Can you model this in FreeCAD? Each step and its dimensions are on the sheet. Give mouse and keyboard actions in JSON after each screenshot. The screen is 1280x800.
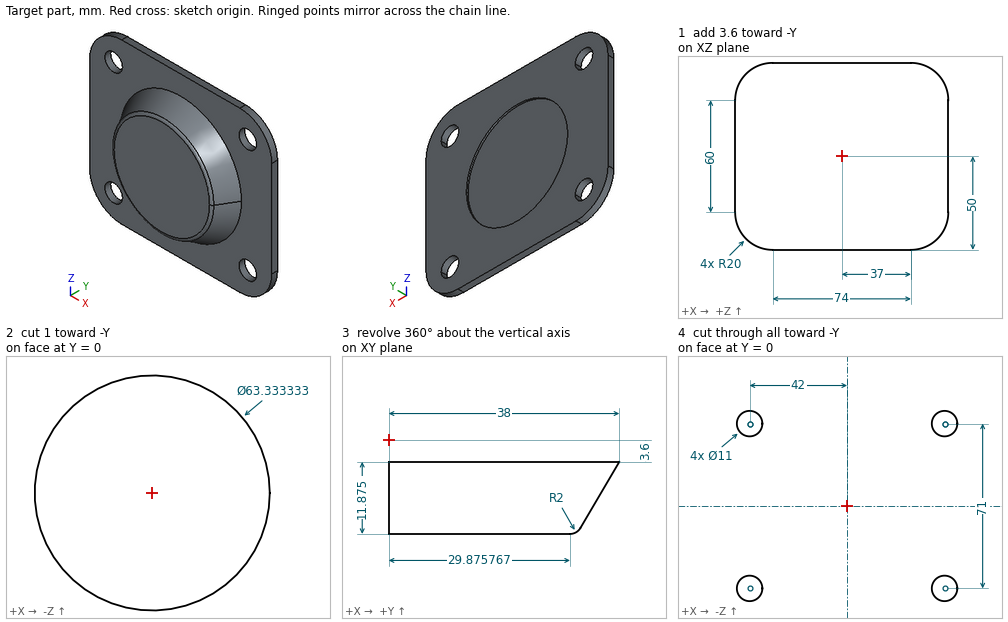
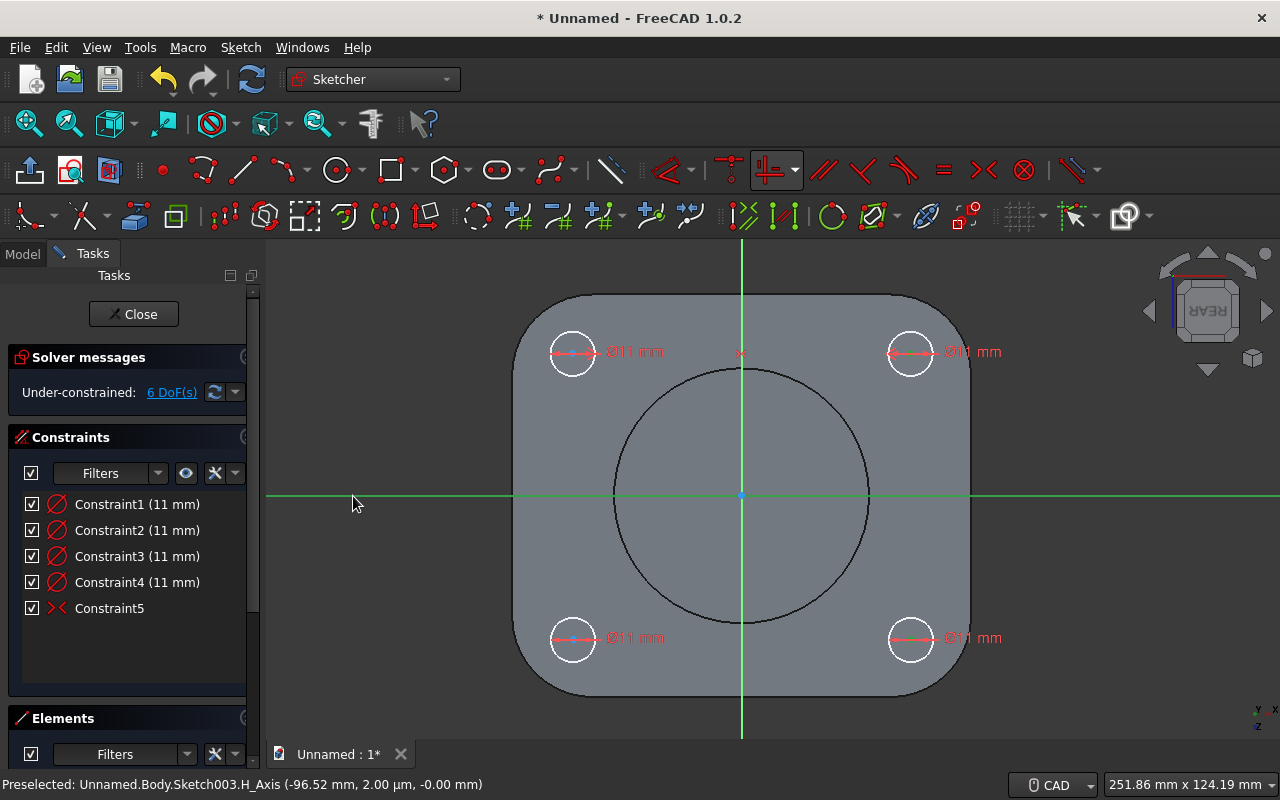
{"action": "left_click", "coordinate": [984, 170]}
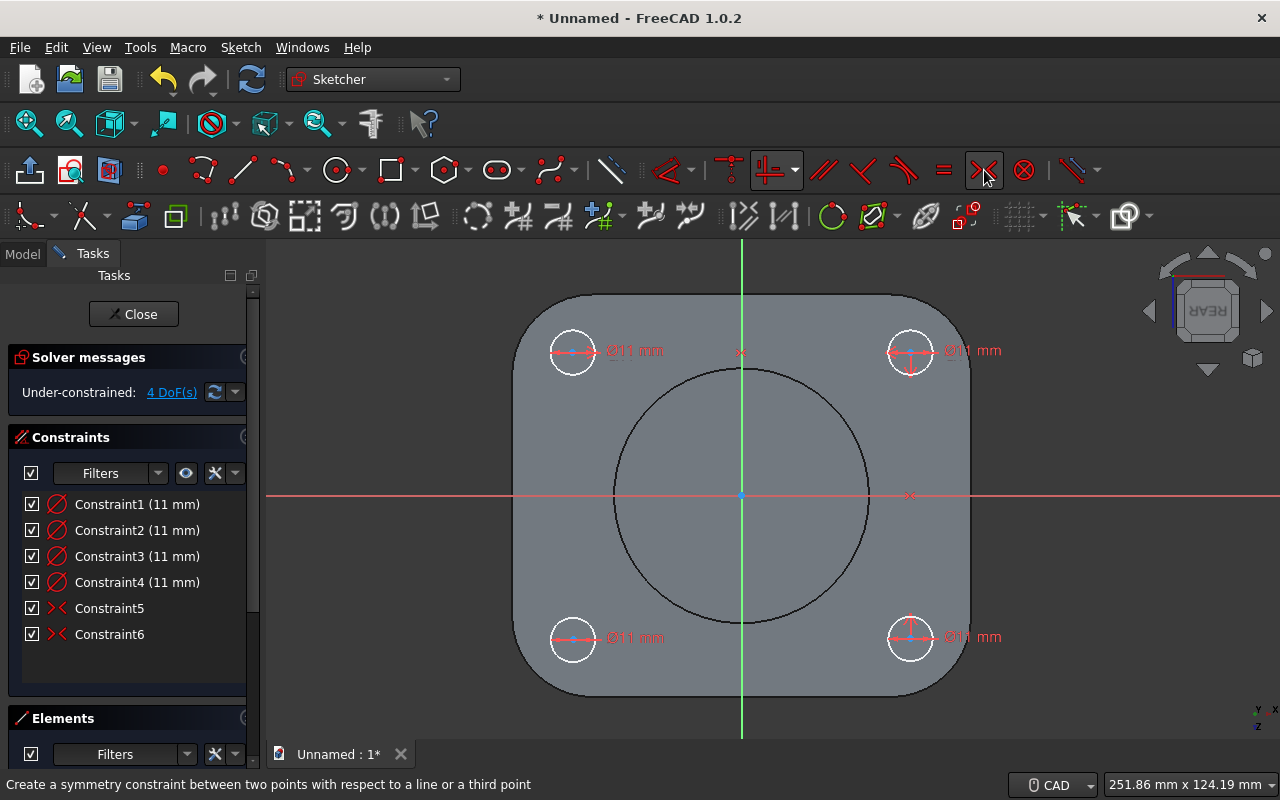
{"action": "left_click", "coordinate": [573, 353]}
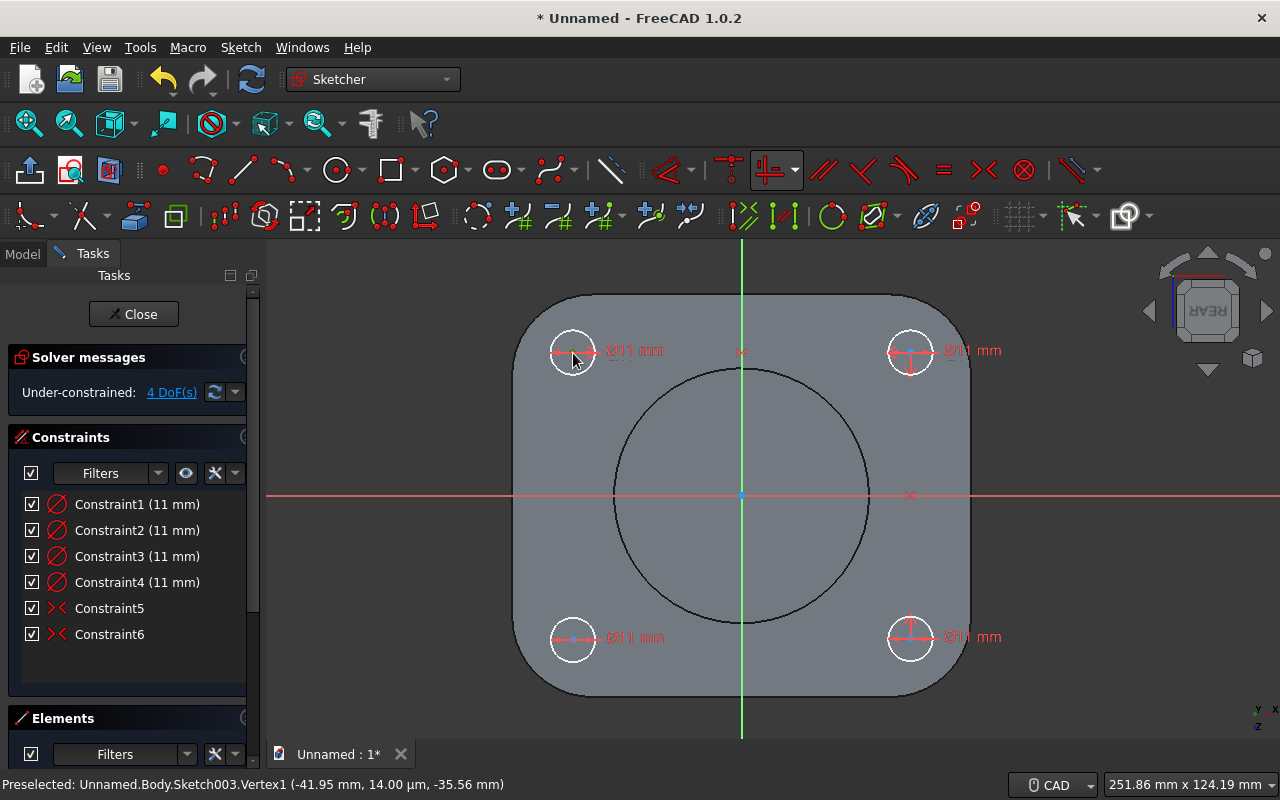
{"action": "left_click", "coordinate": [573, 640]}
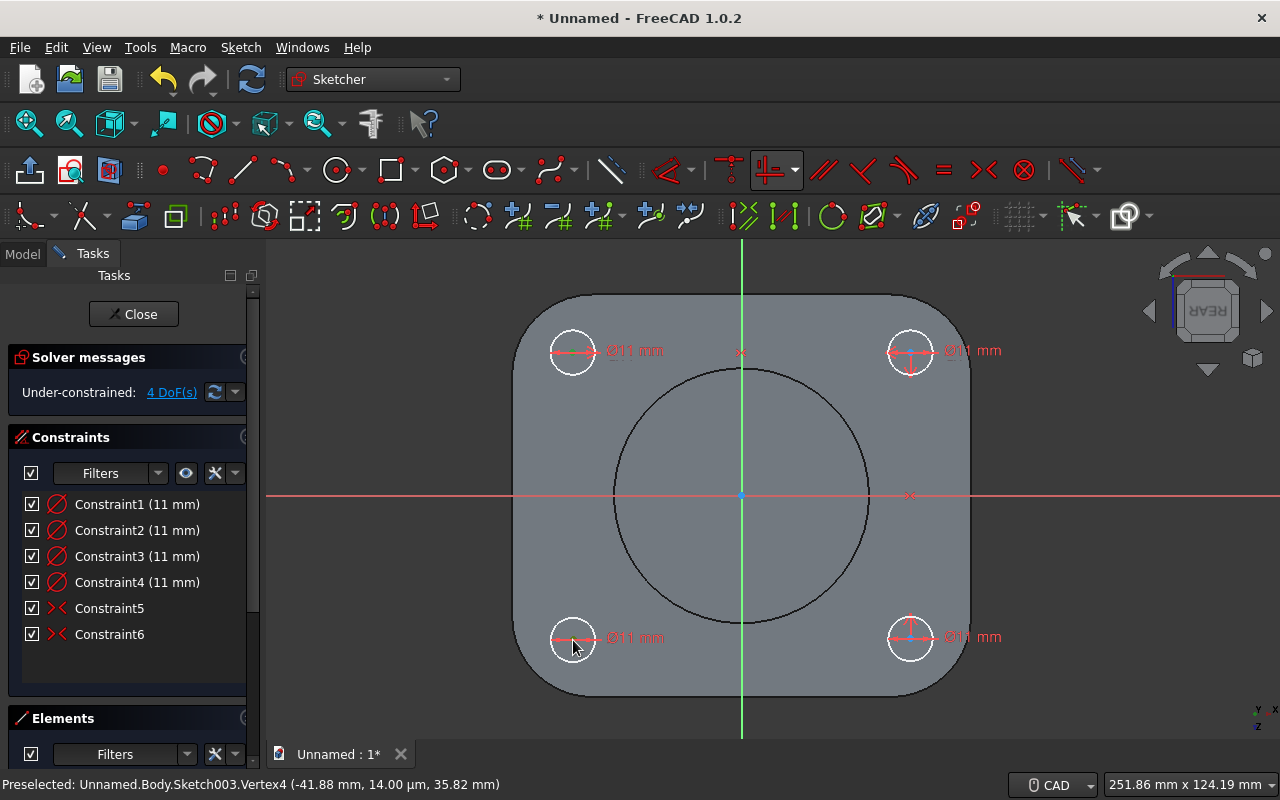
{"action": "left_click", "coordinate": [353, 496]}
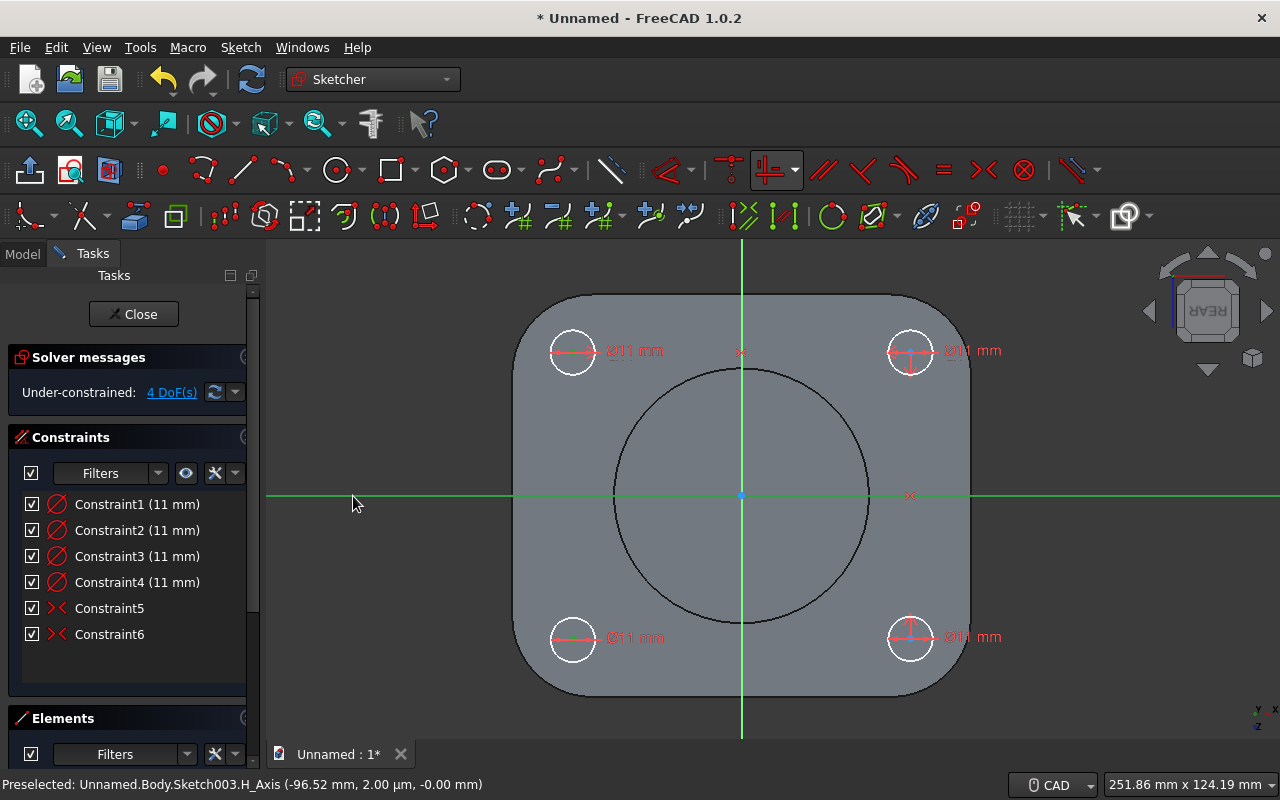
{"action": "left_click", "coordinate": [984, 170]}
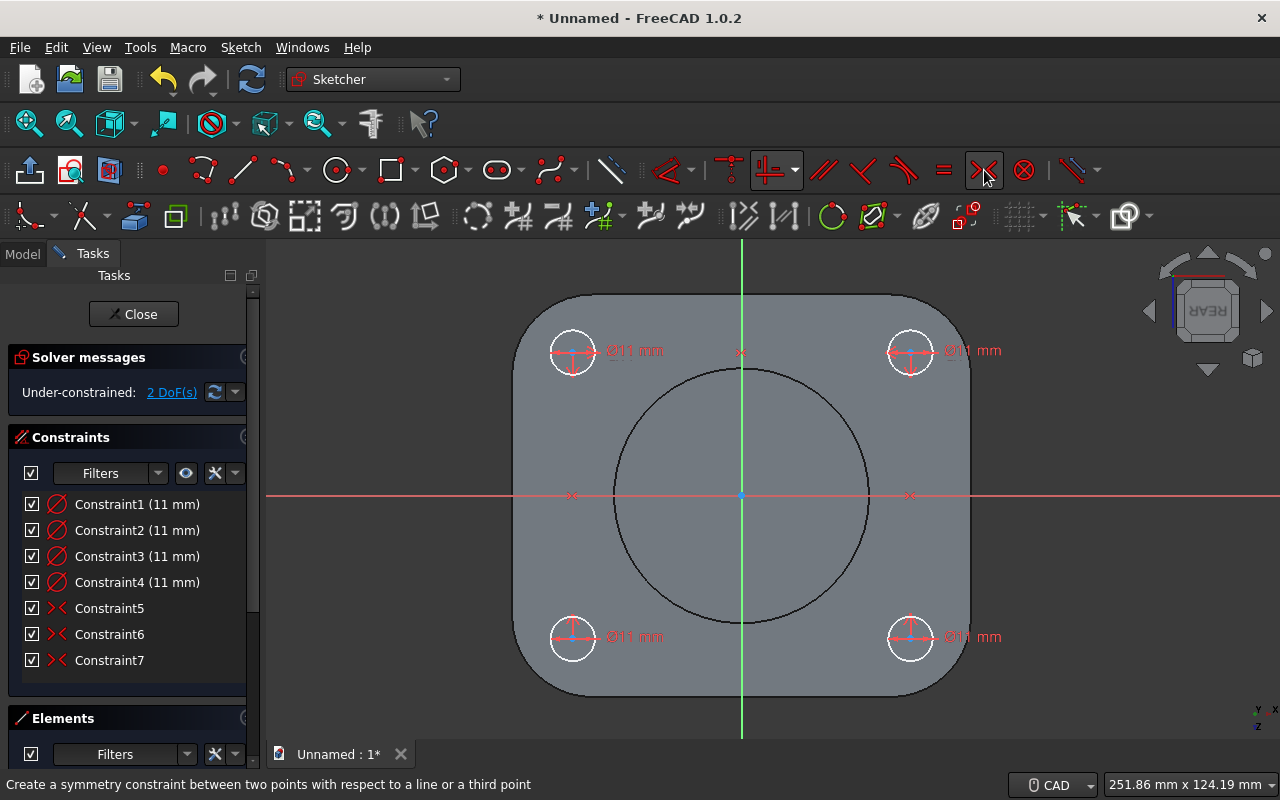
{"action": "left_click", "coordinate": [666, 170]}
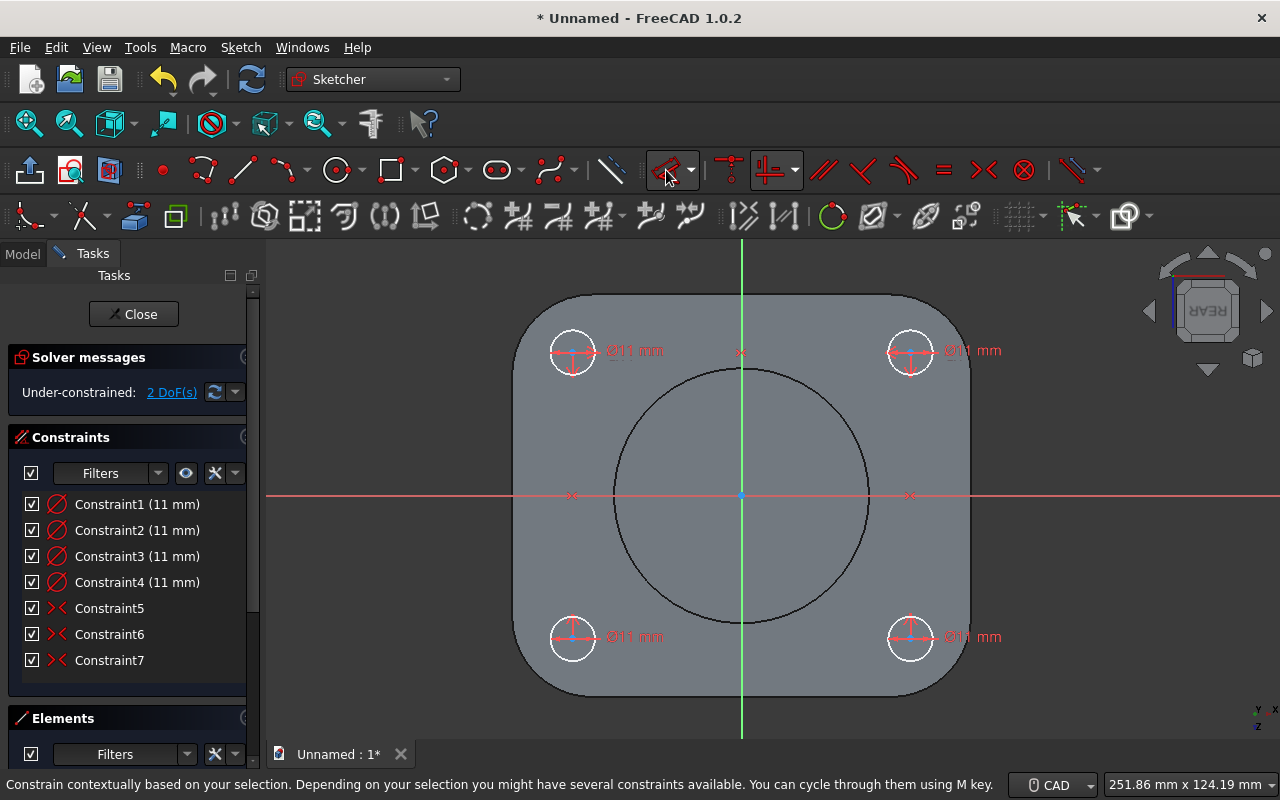
{"action": "left_click", "coordinate": [573, 353]}
{"action": "left_click", "coordinate": [657, 319]}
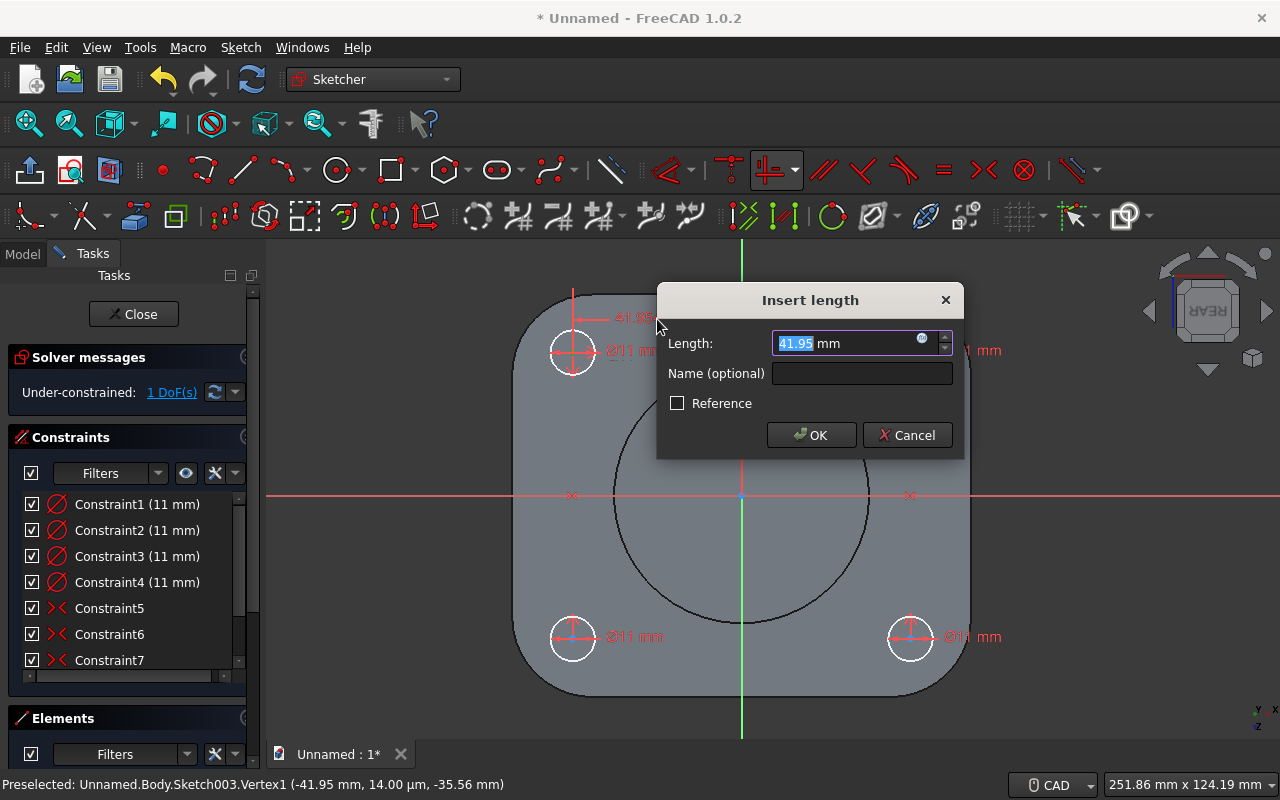
{"action": "type", "text": "42"}
{"action": "key", "text": "Return"}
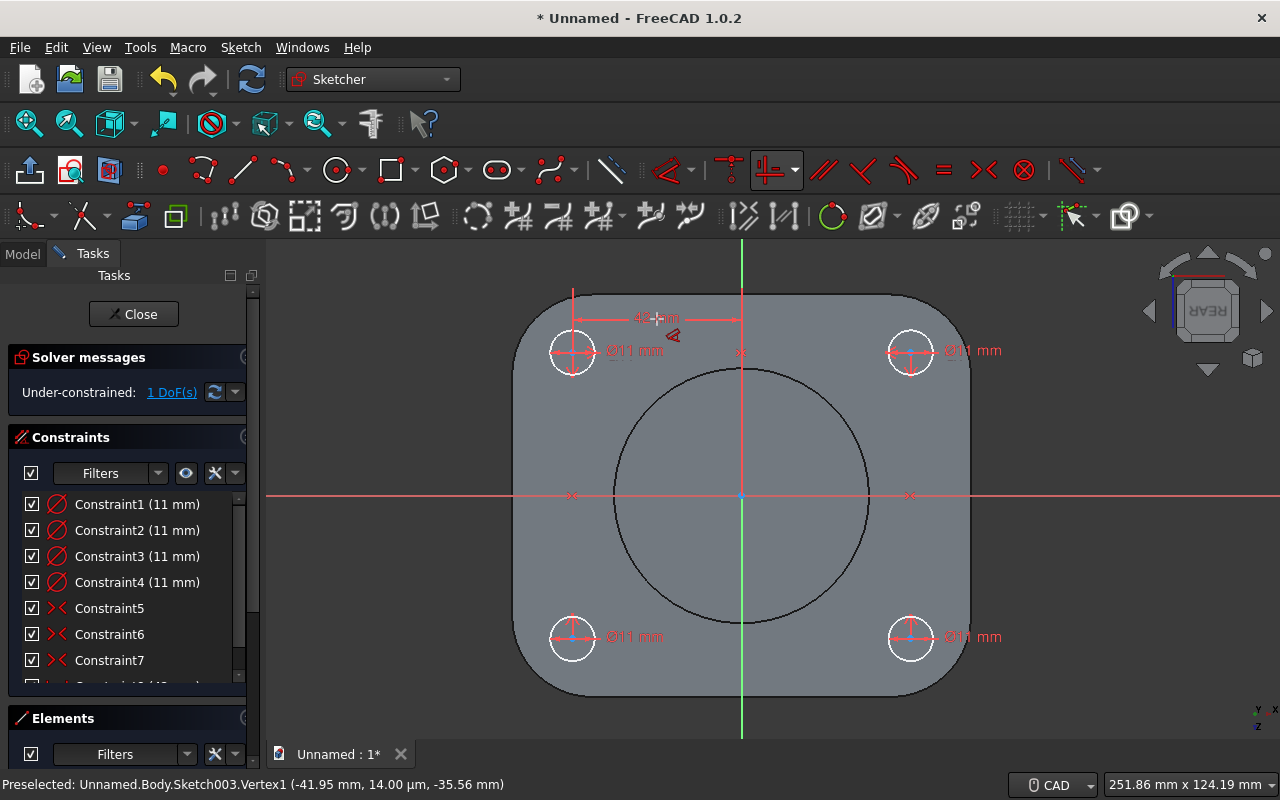
{"action": "left_click", "coordinate": [911, 353]}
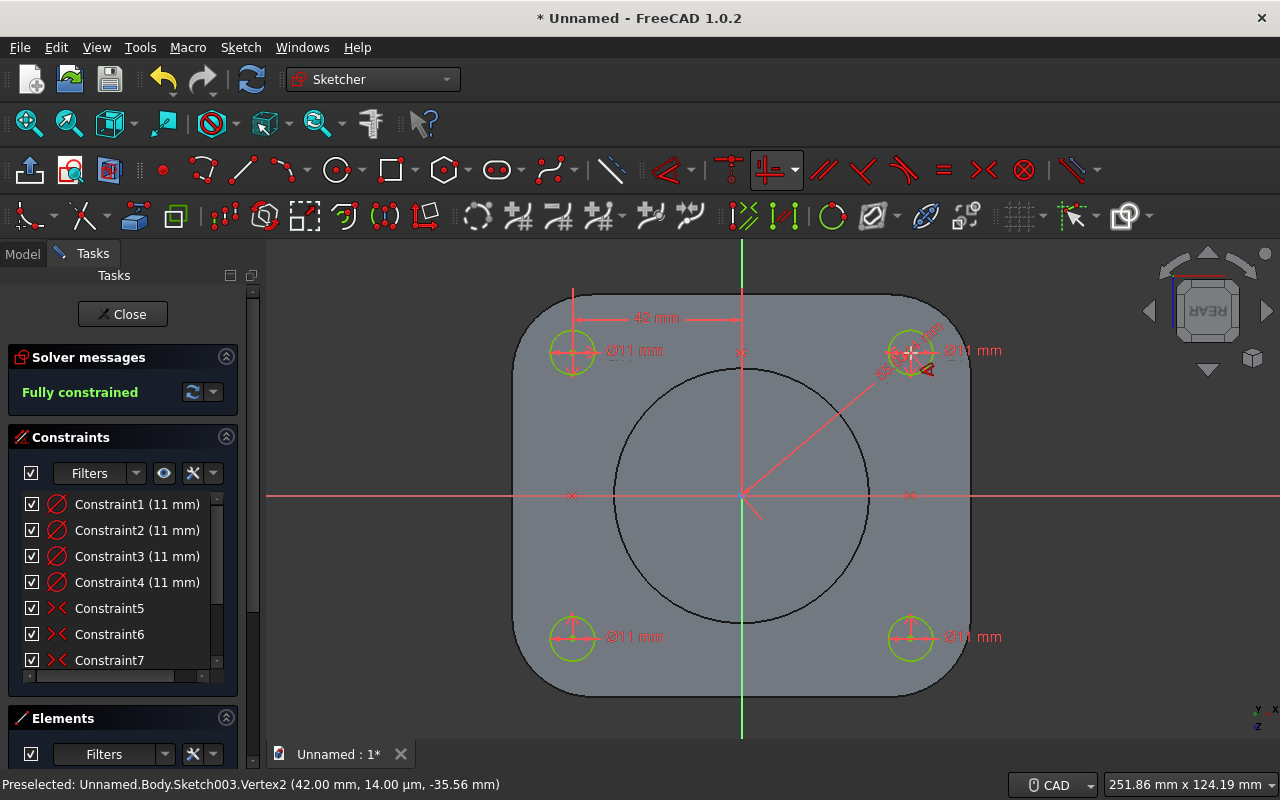
{"action": "left_click", "coordinate": [911, 639]}
{"action": "left_click", "coordinate": [945, 430]}